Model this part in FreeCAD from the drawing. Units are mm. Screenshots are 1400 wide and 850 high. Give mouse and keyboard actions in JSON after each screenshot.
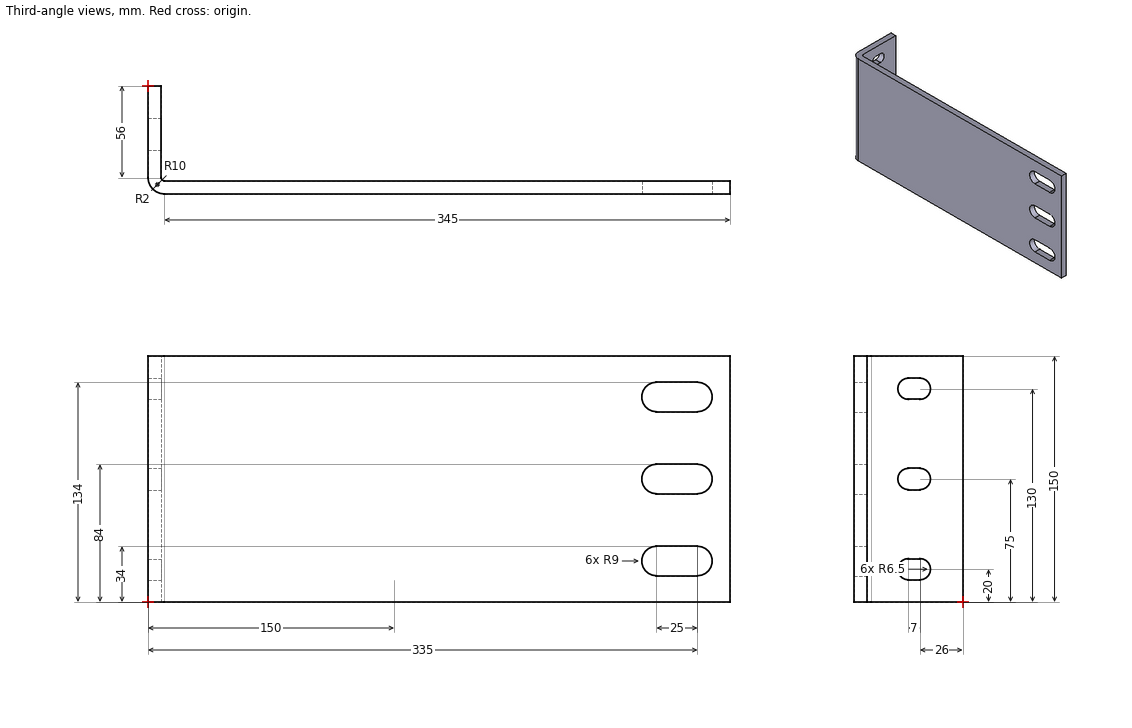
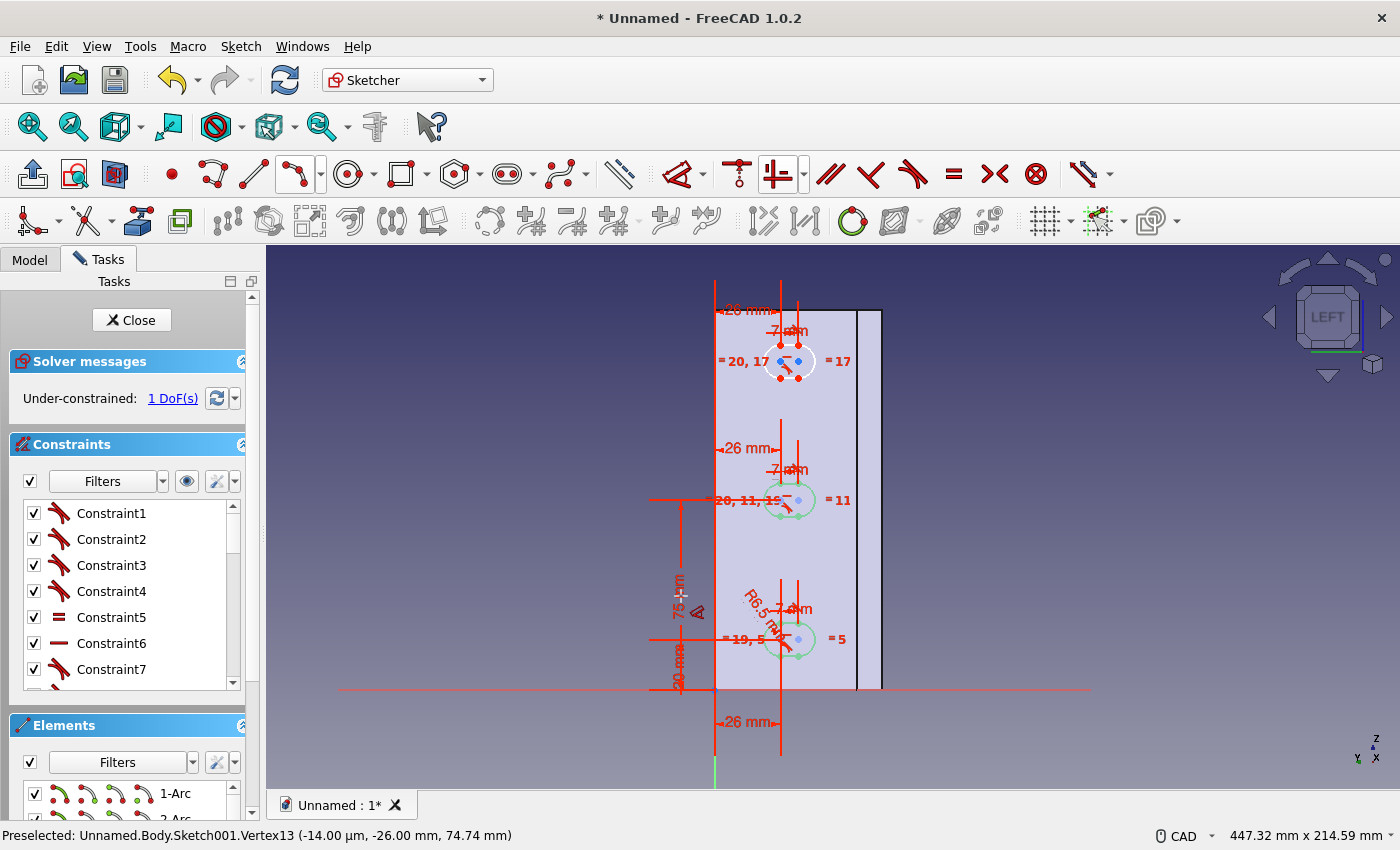
{"action": "left_click", "coordinate": [781, 362]}
{"action": "left_click", "coordinate": [681, 526]}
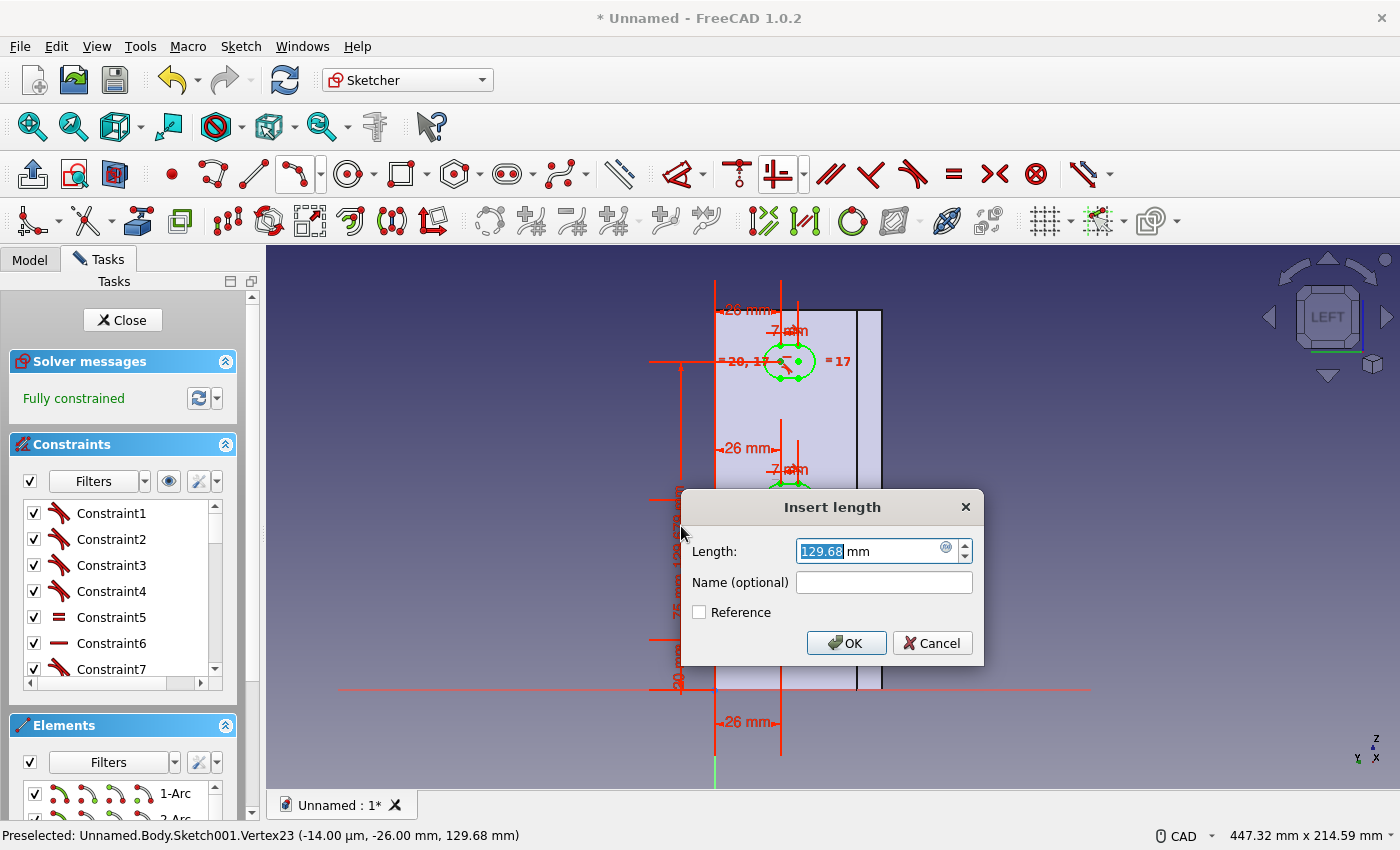
{"action": "type", "text": "130"}
{"action": "key", "text": "Return"}
{"action": "key", "text": "Escape"}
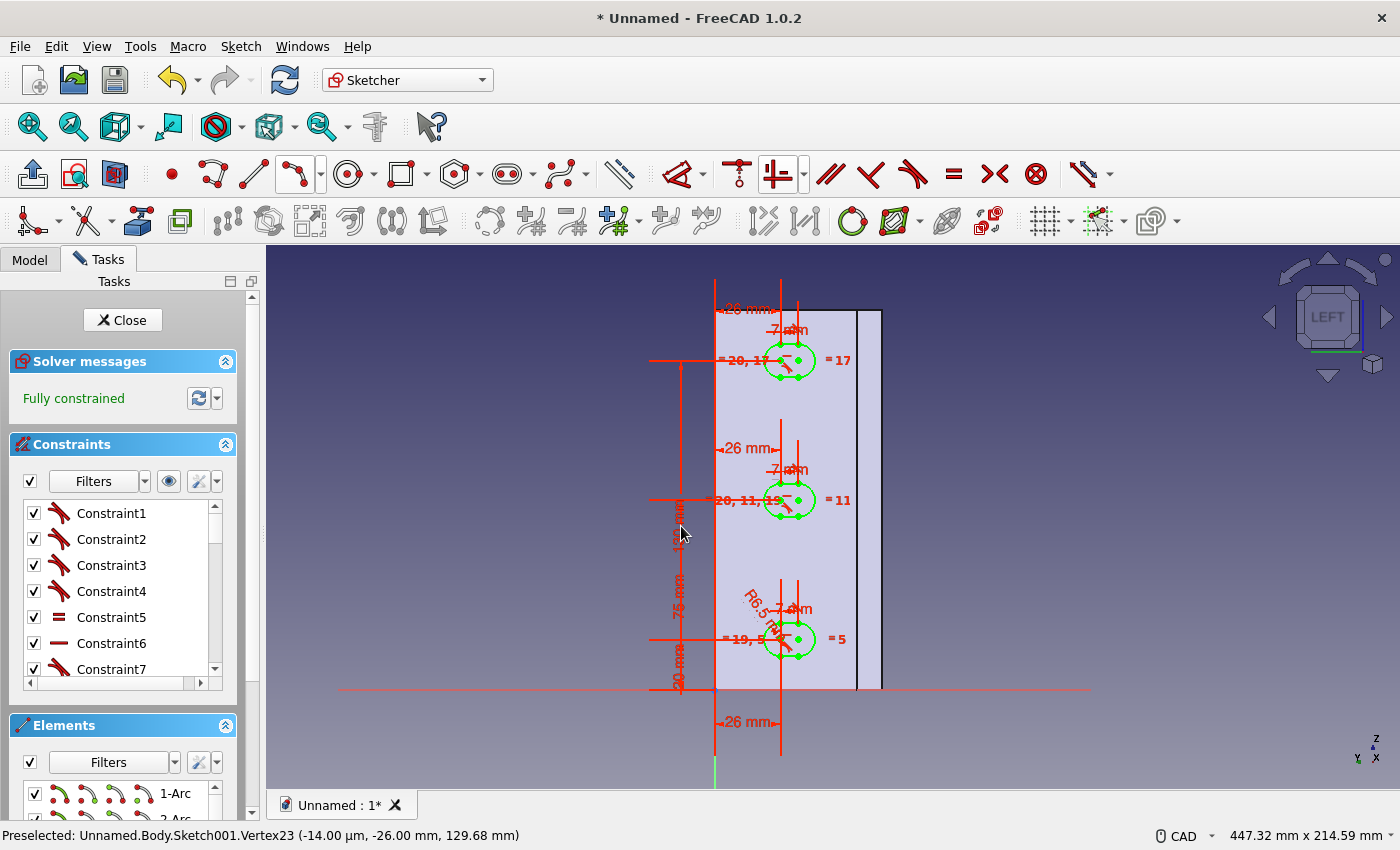
{"action": "left_click", "coordinate": [123, 320]}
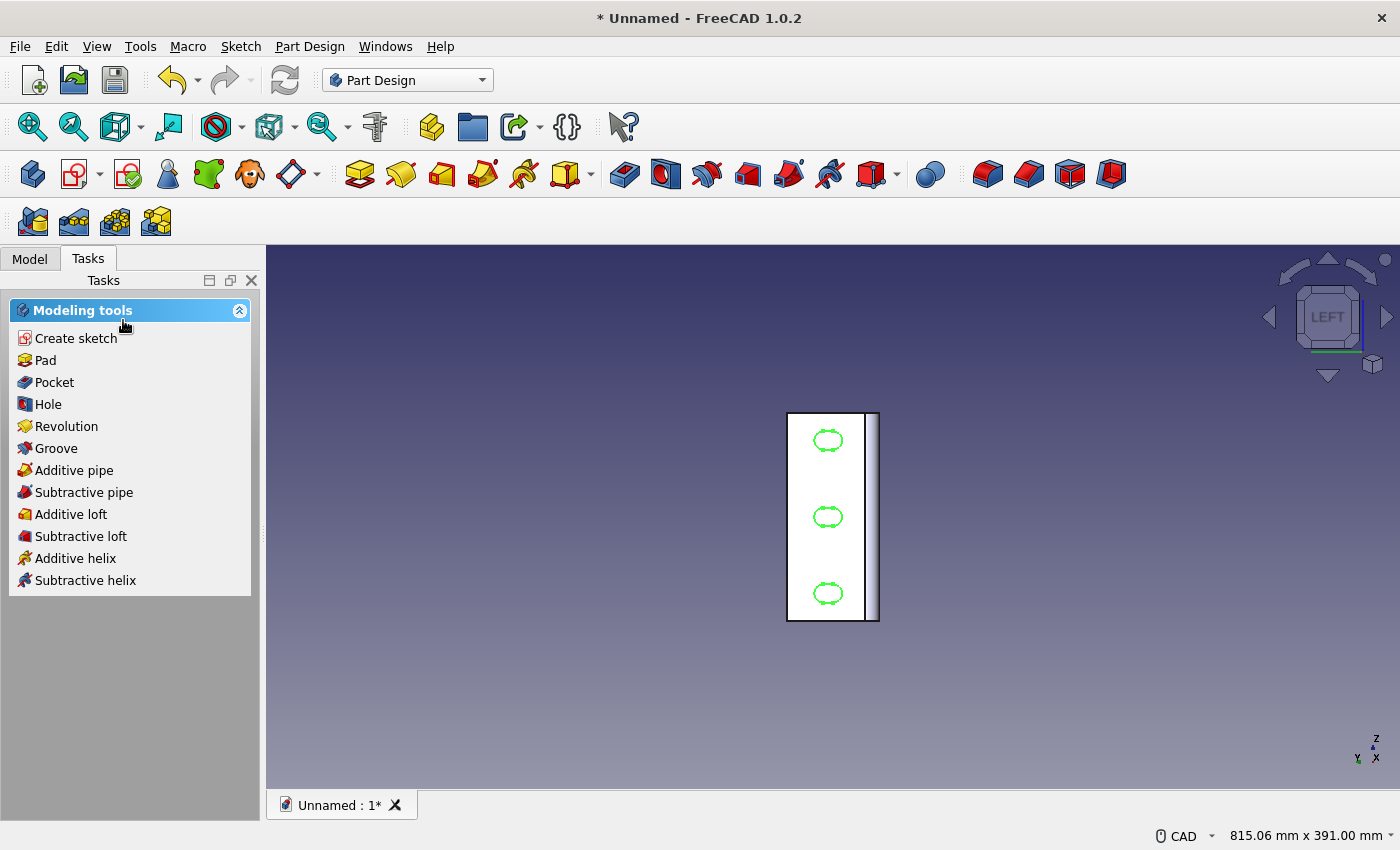
{"action": "left_click", "coordinate": [625, 174]}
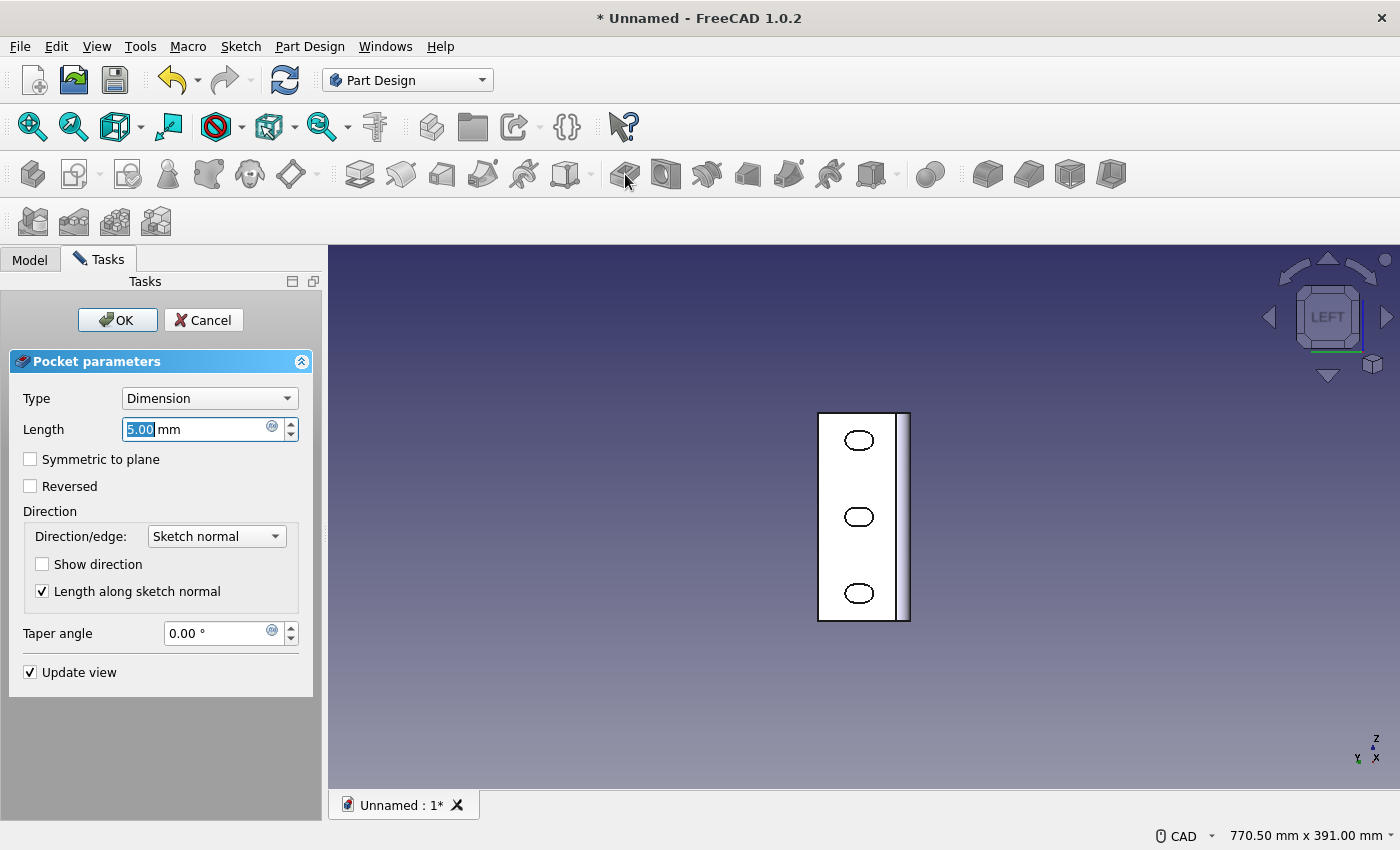
{"action": "type", "text": "150"}
{"action": "key", "text": "Tab"}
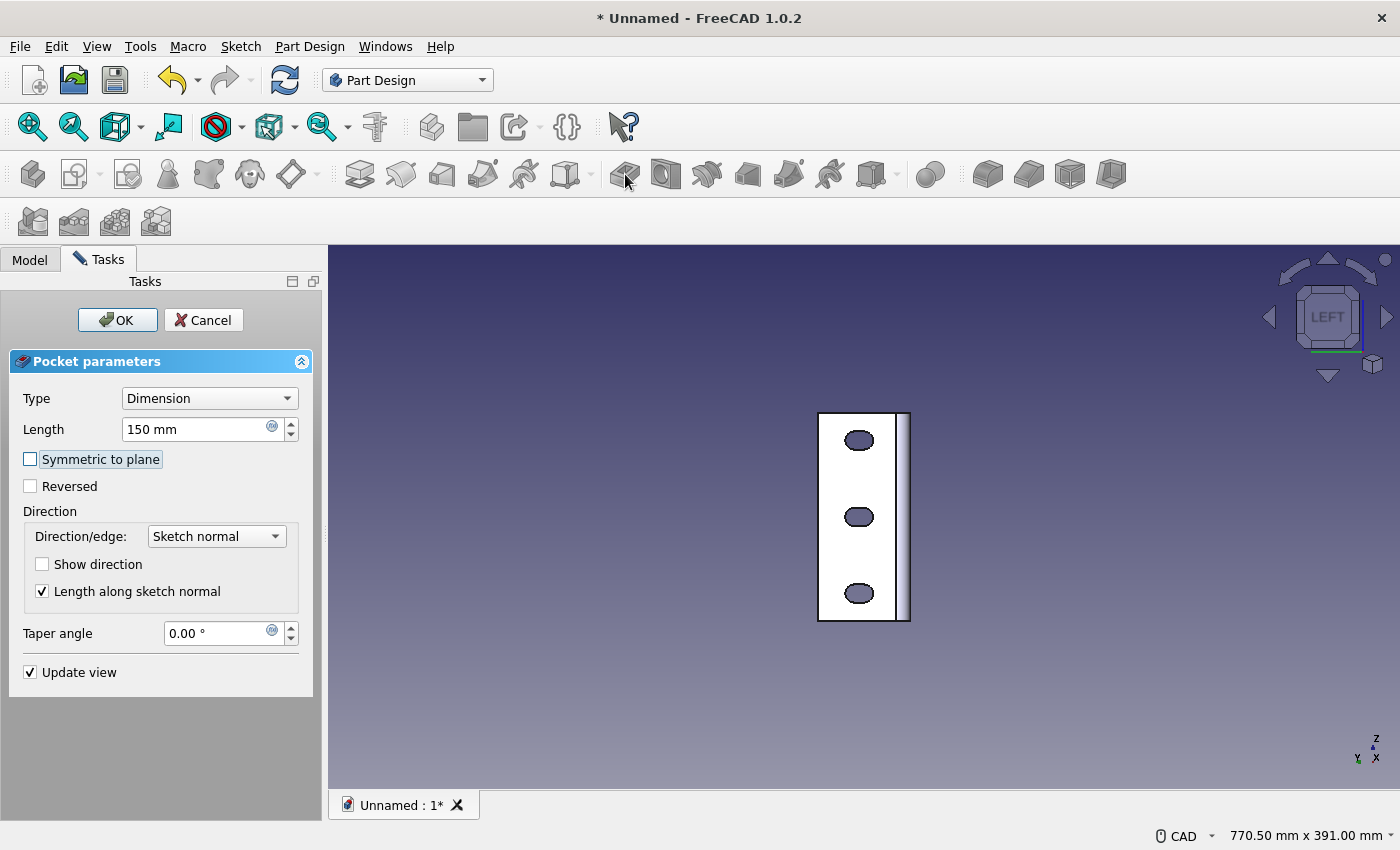
{"action": "left_click", "coordinate": [118, 320]}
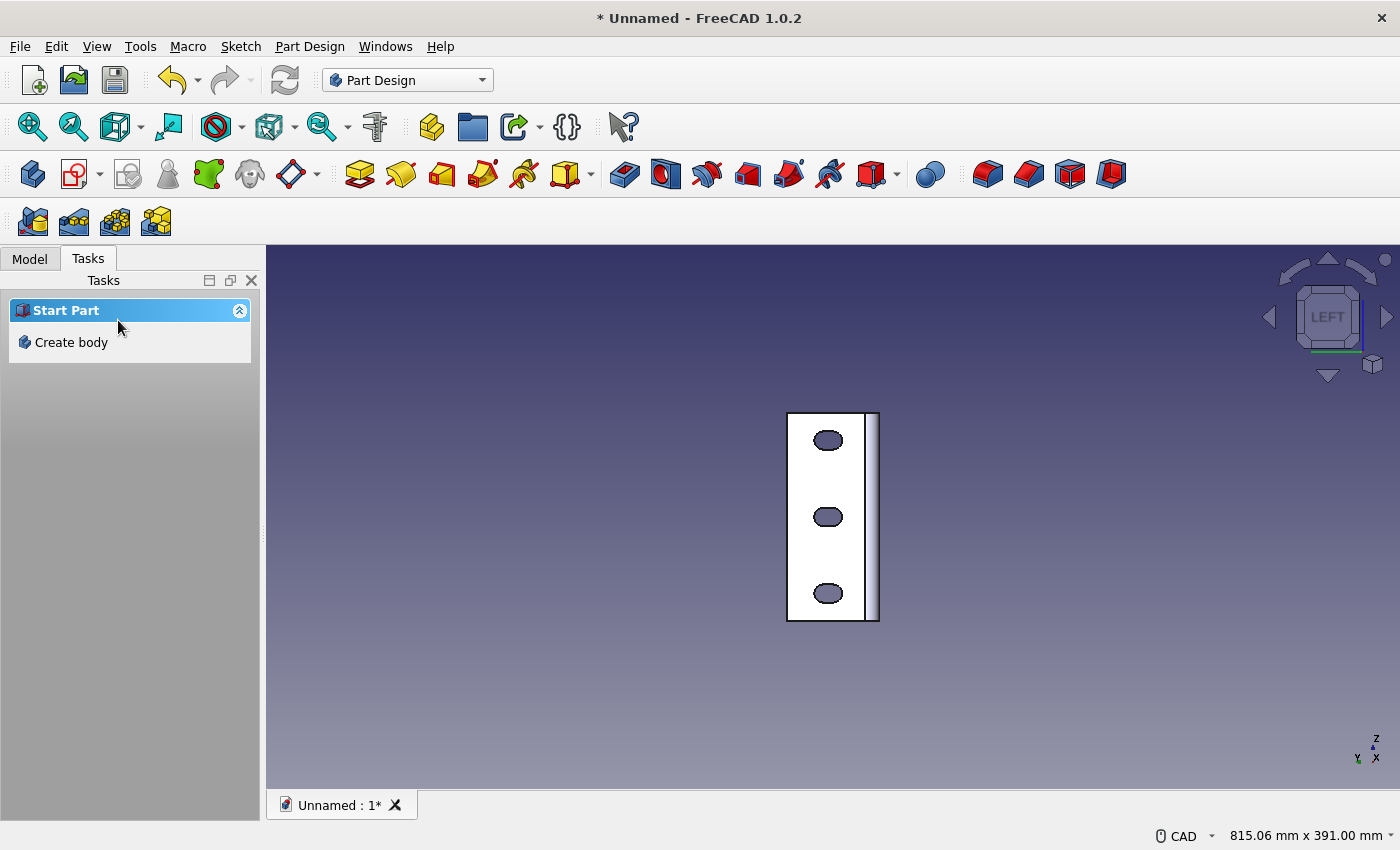
{"action": "left_click", "coordinate": [33, 128]}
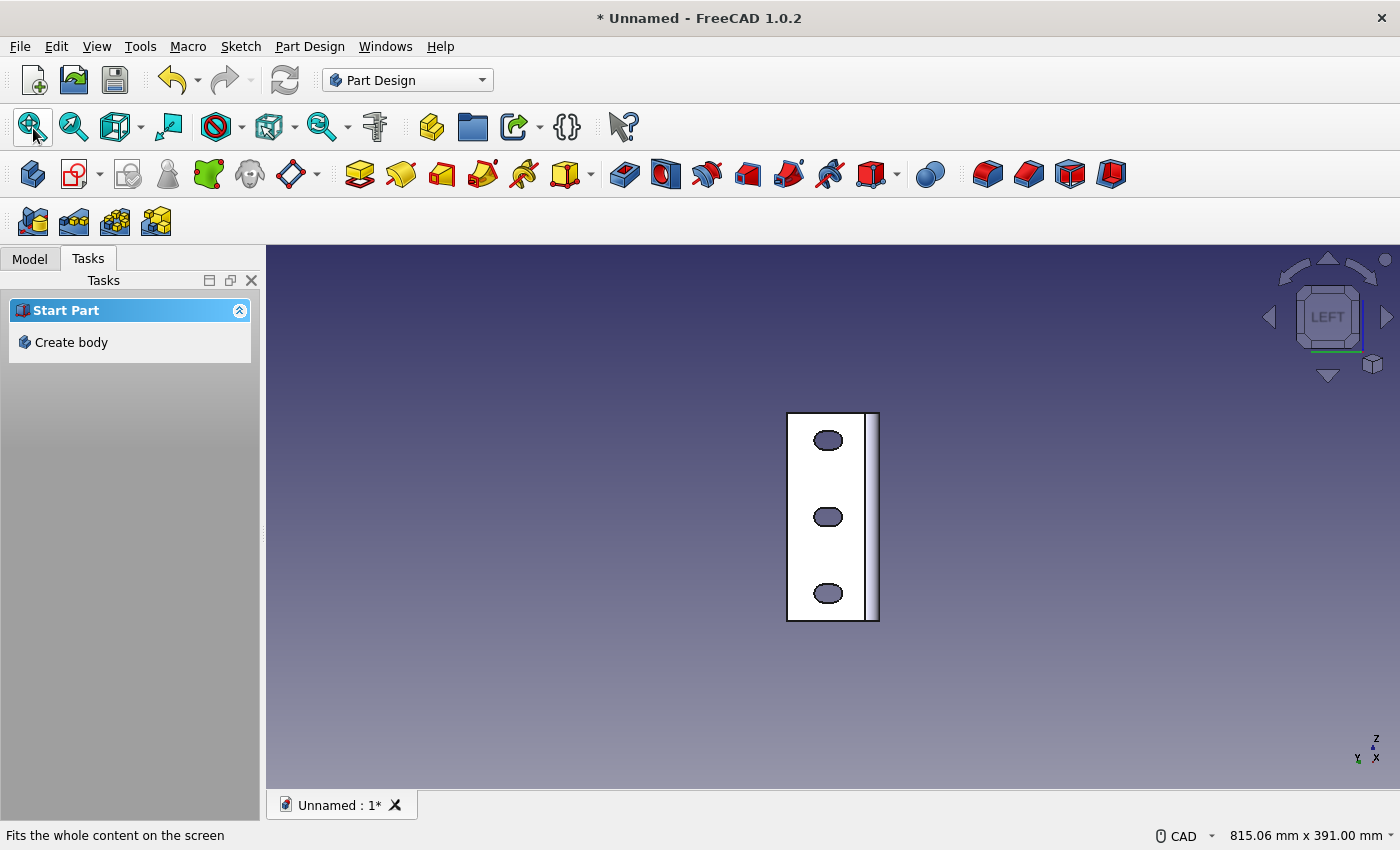
{"action": "key", "text": "4"}